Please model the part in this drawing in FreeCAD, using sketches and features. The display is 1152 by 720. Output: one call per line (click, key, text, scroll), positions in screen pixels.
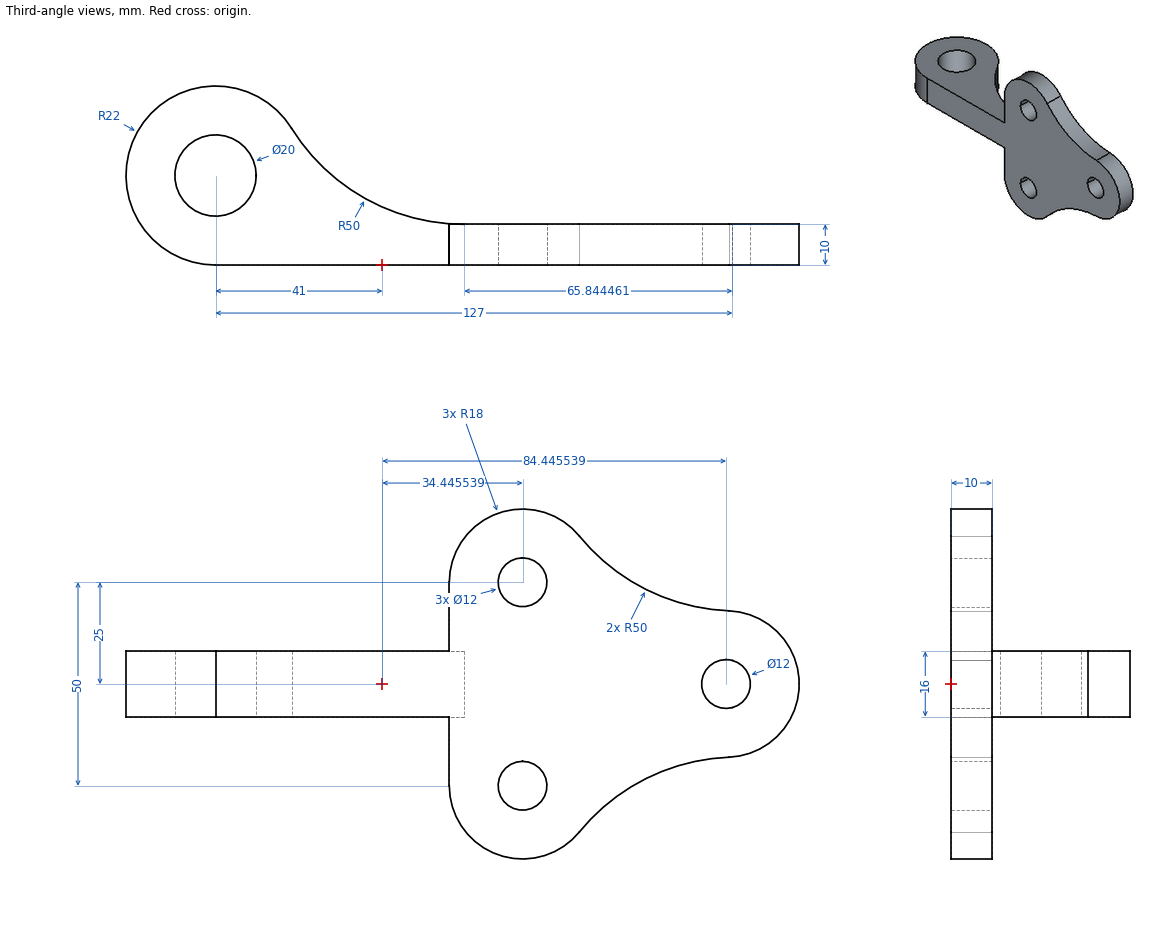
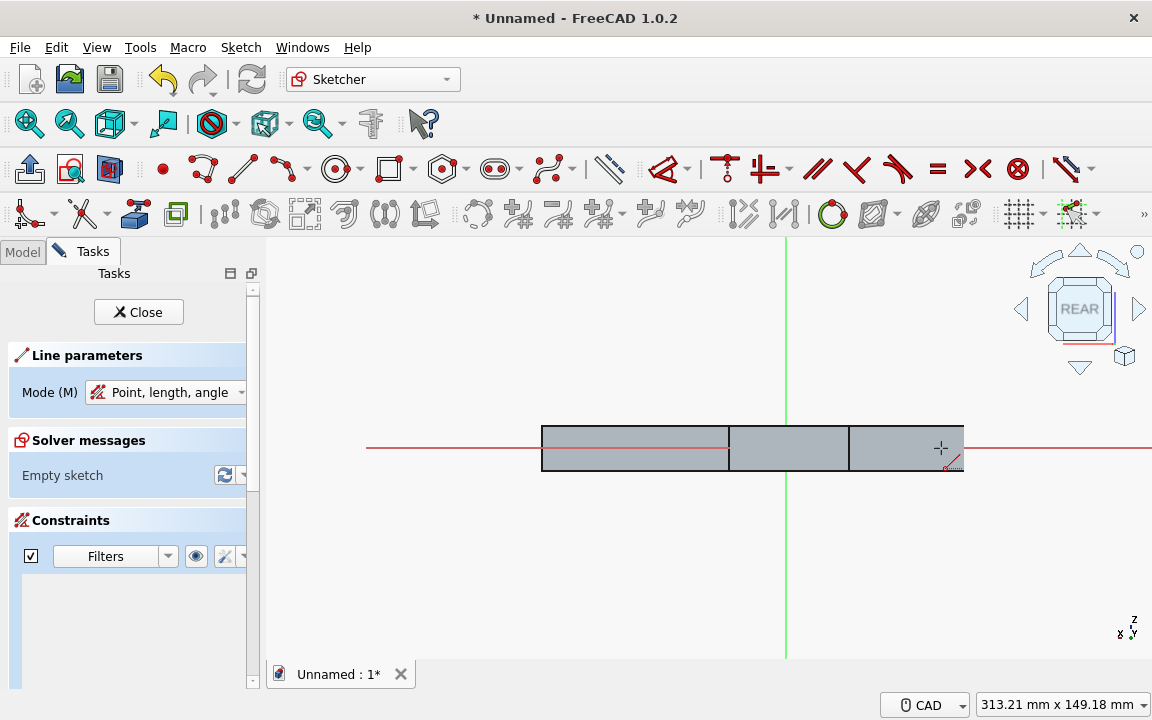
click(739, 519)
click(739, 377)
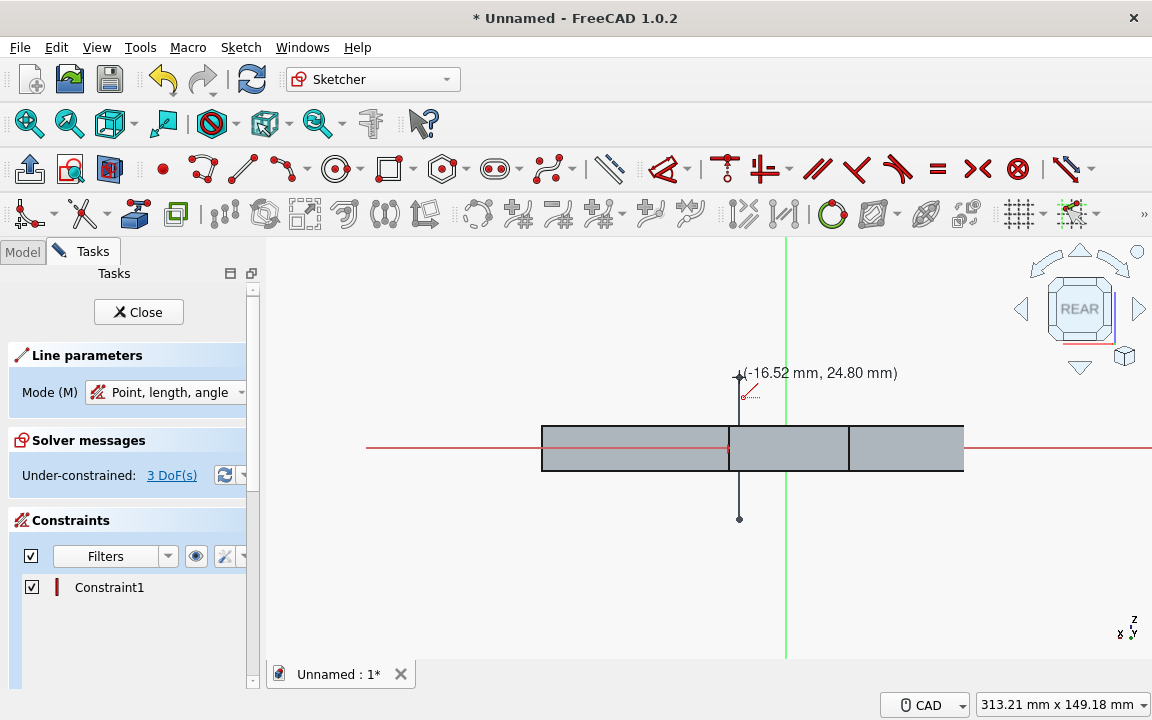
key(g)
key(3)
key(a)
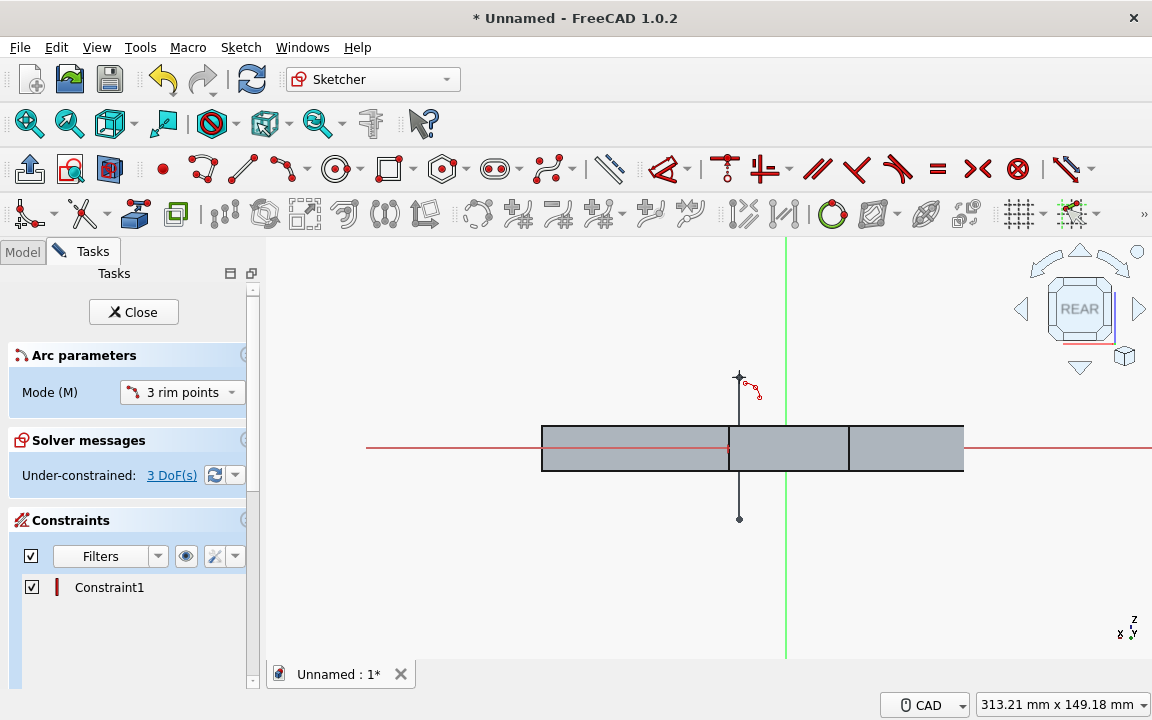
click(739, 378)
click(649, 345)
click(705, 329)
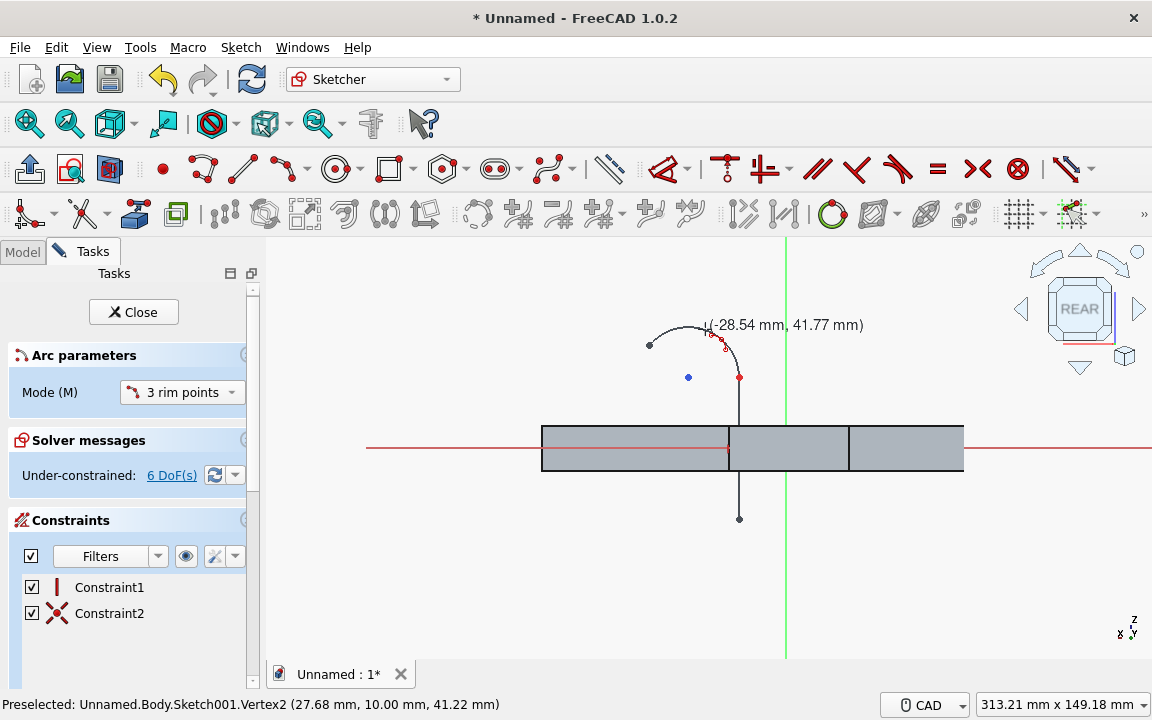
click(649, 346)
click(545, 397)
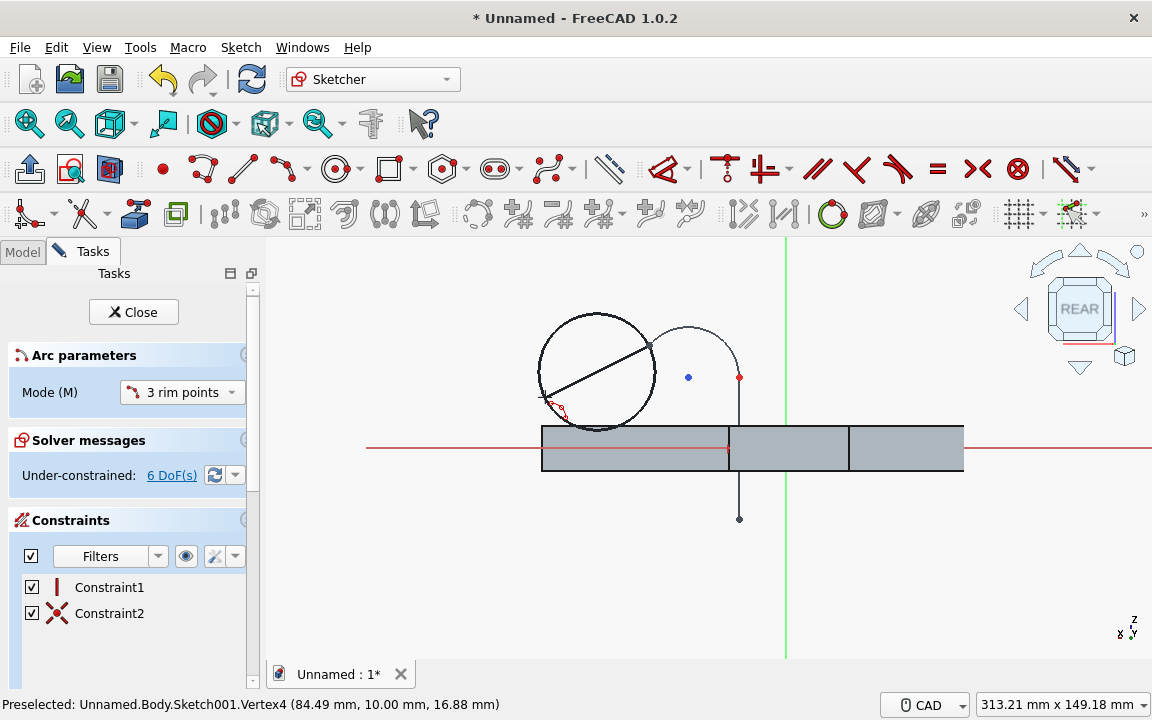
scroll(602, 382, up, 2)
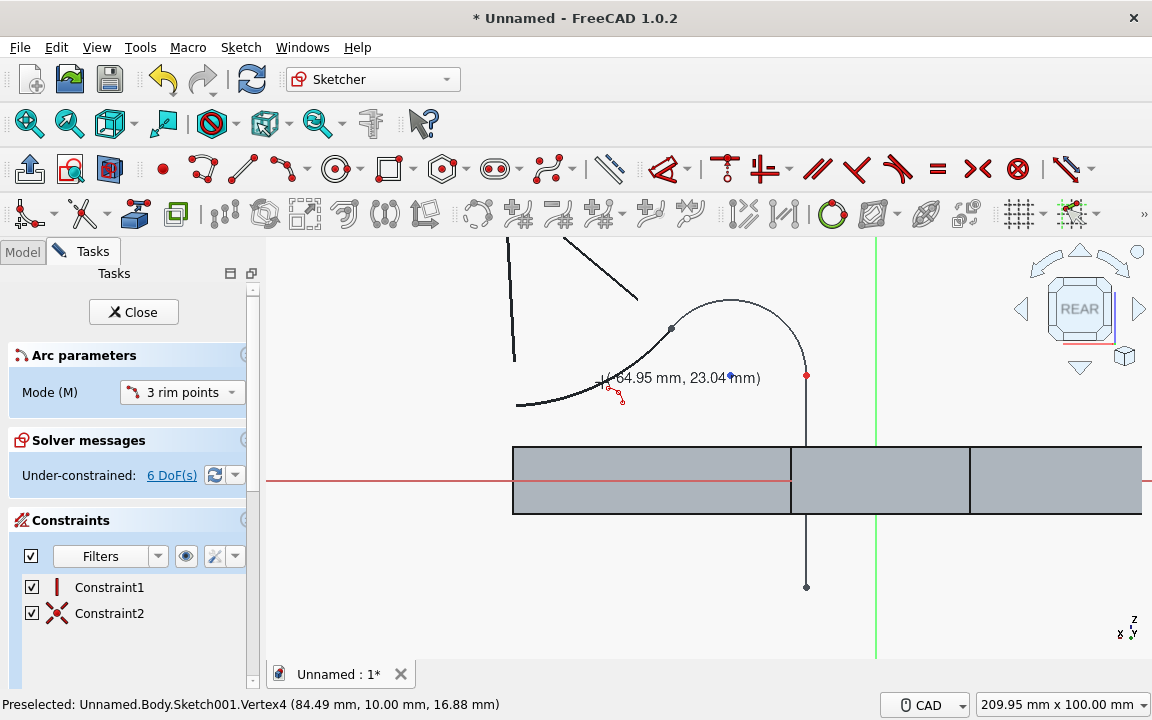
click(602, 383)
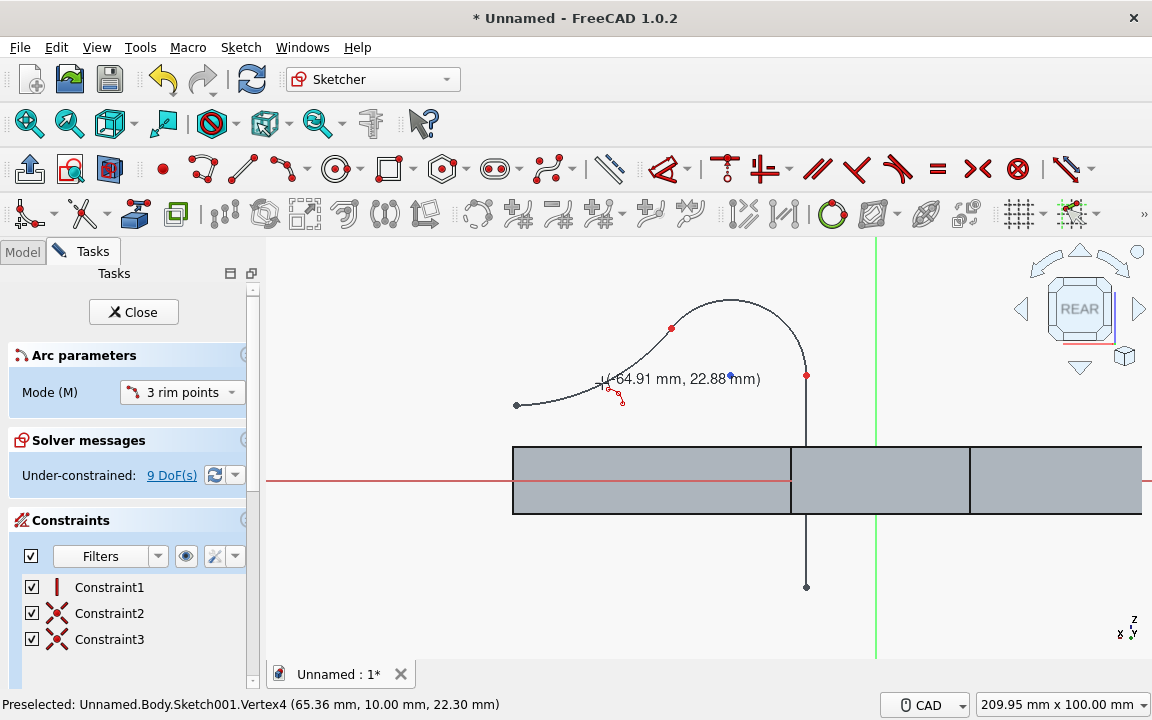
click(517, 406)
click(517, 556)
click(447, 458)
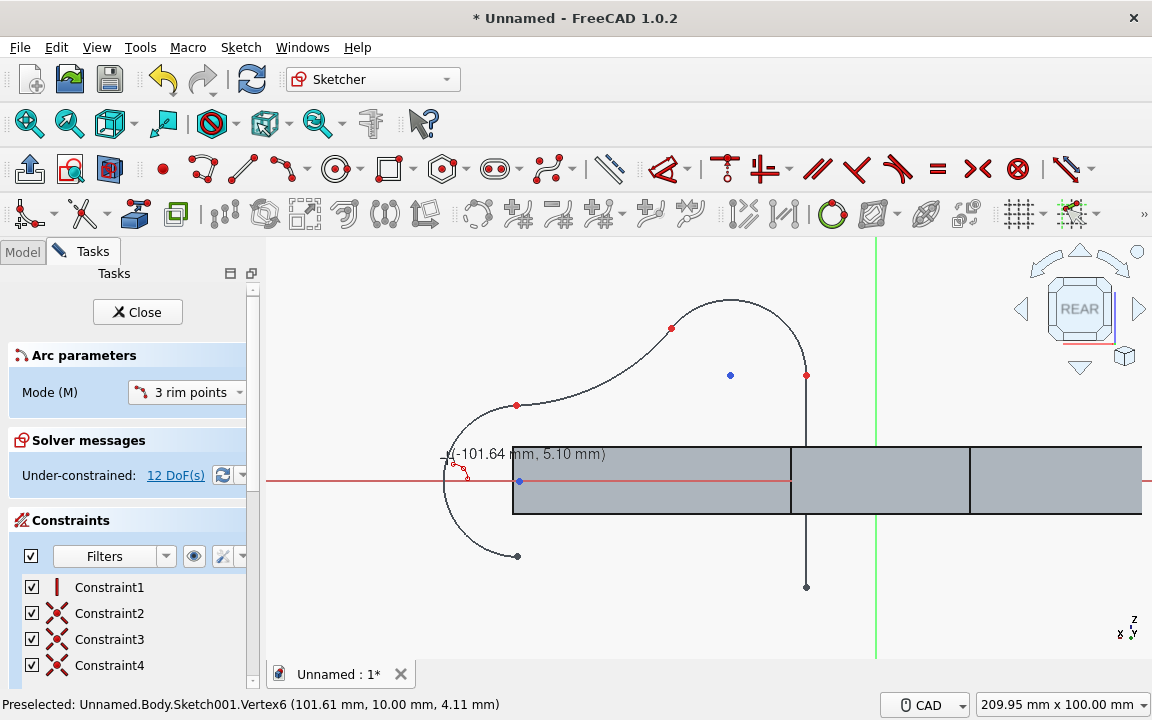
click(517, 557)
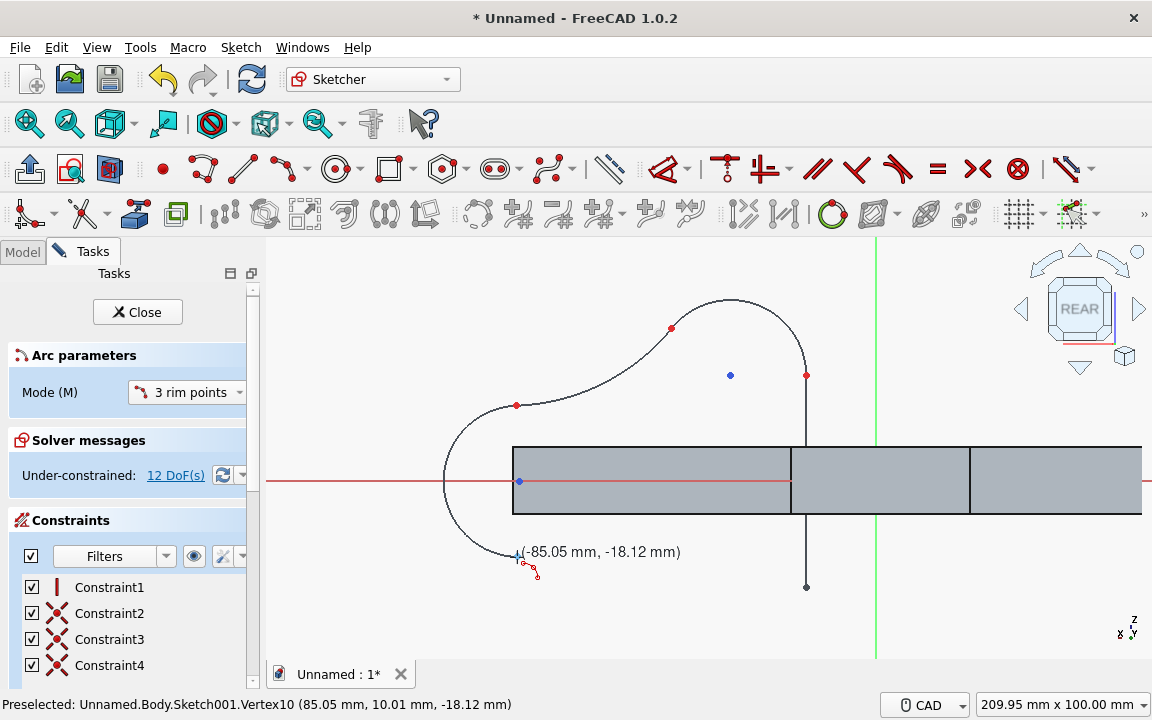
scroll(601, 382, down, 2)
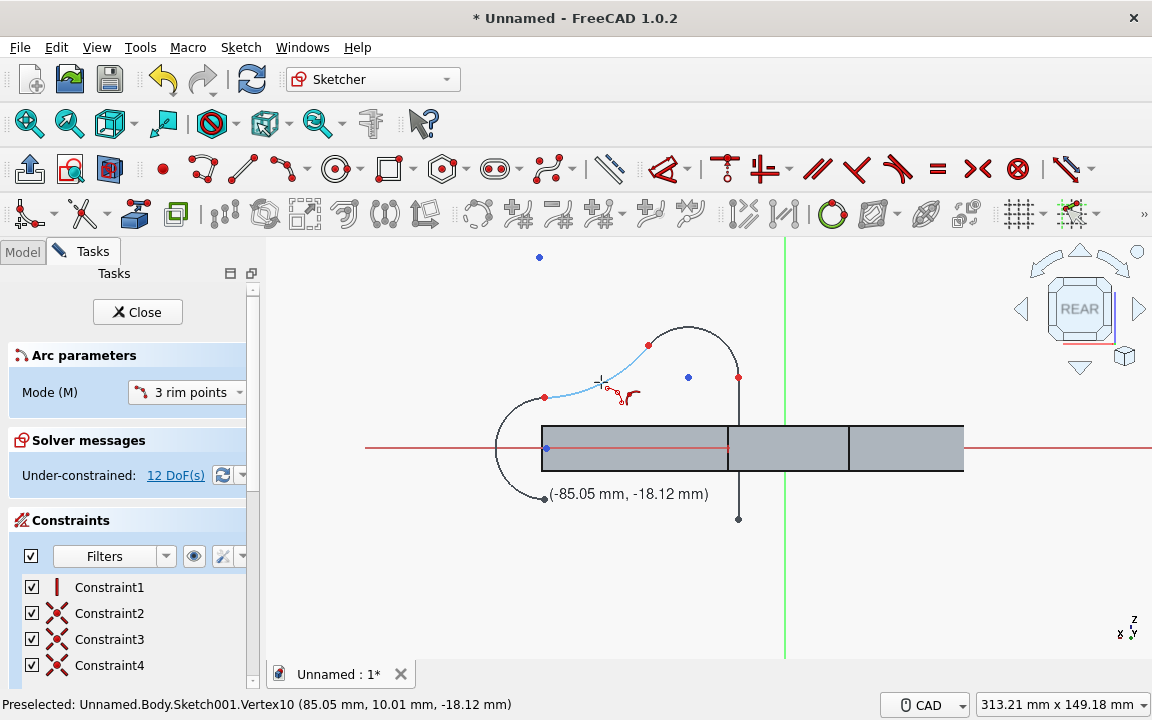
click(648, 551)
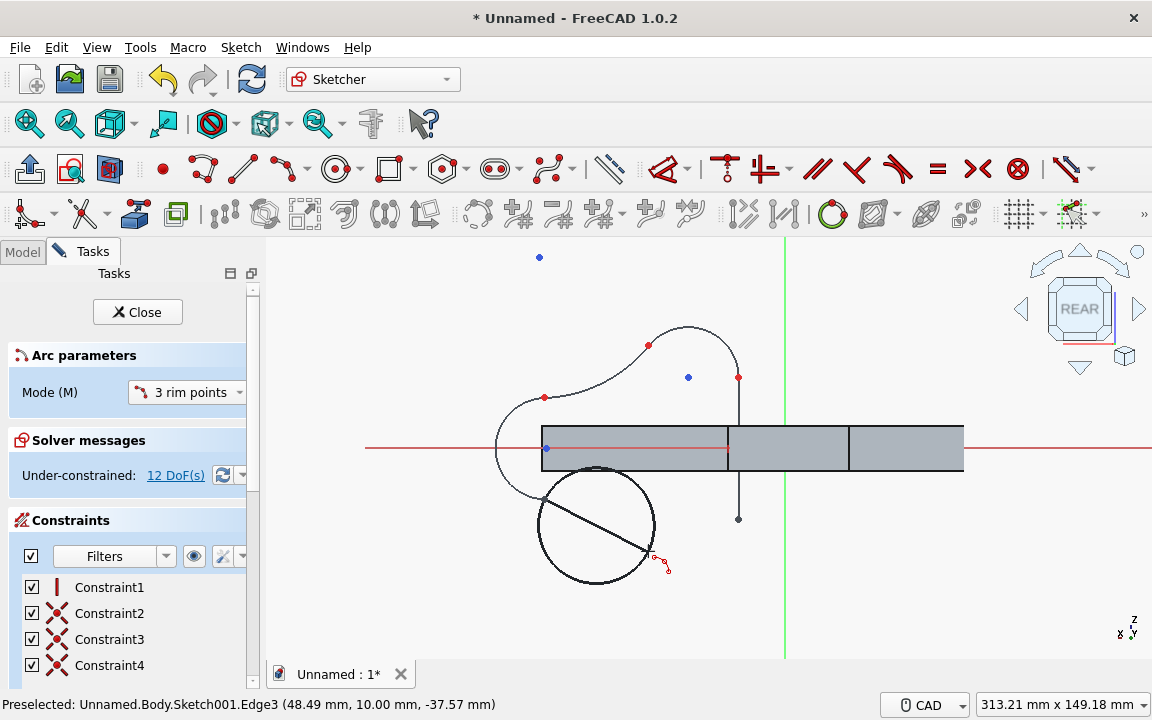
scroll(602, 514, up, 2)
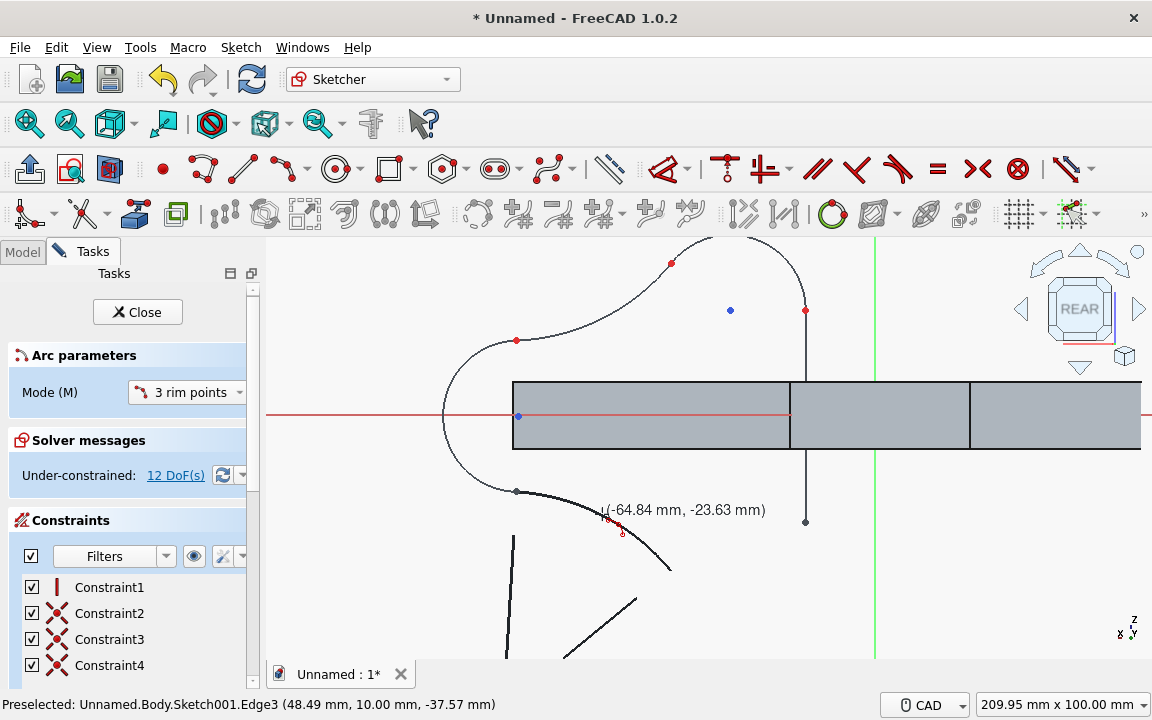
click(602, 513)